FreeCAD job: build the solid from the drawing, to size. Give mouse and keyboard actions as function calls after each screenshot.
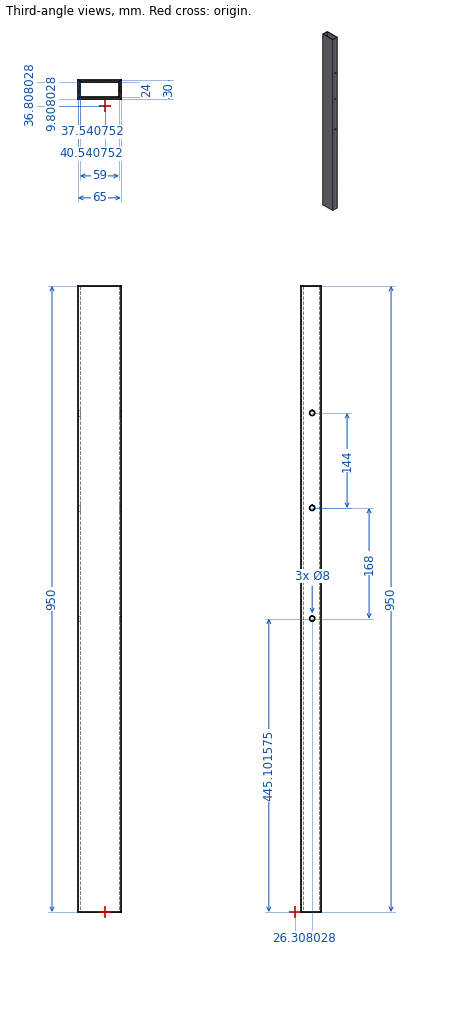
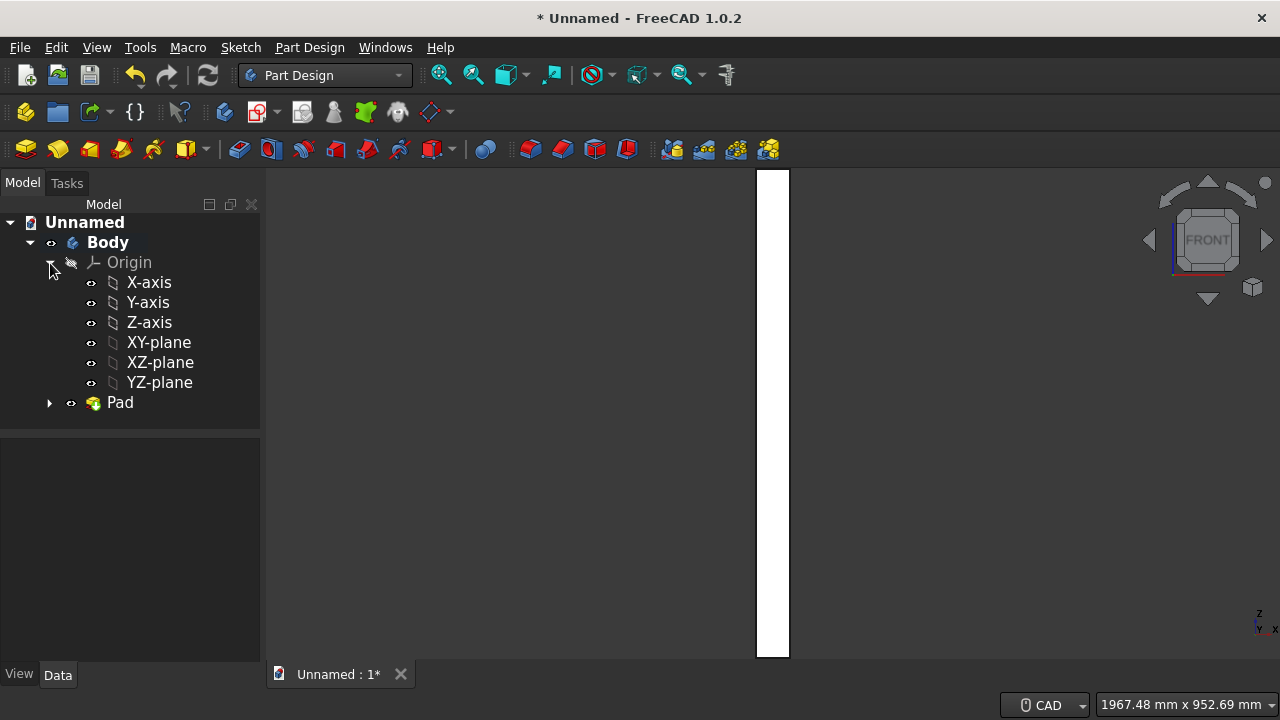
click(136, 343)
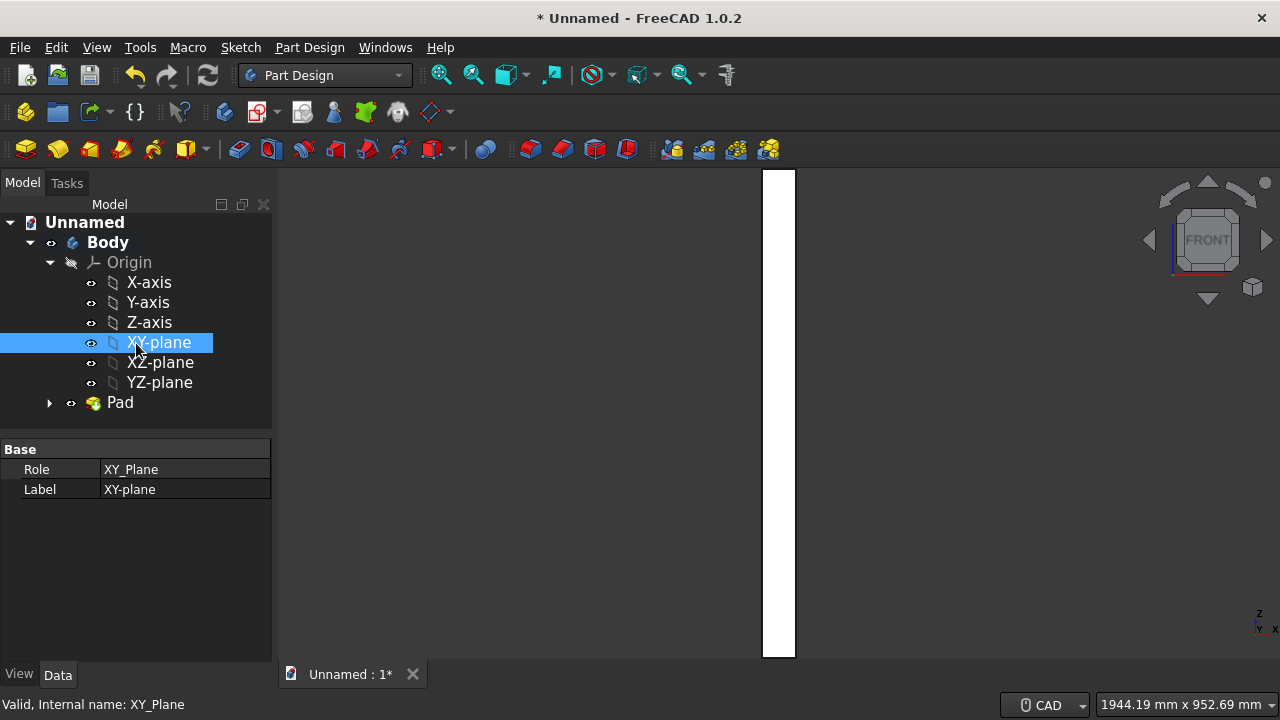
click(430, 112)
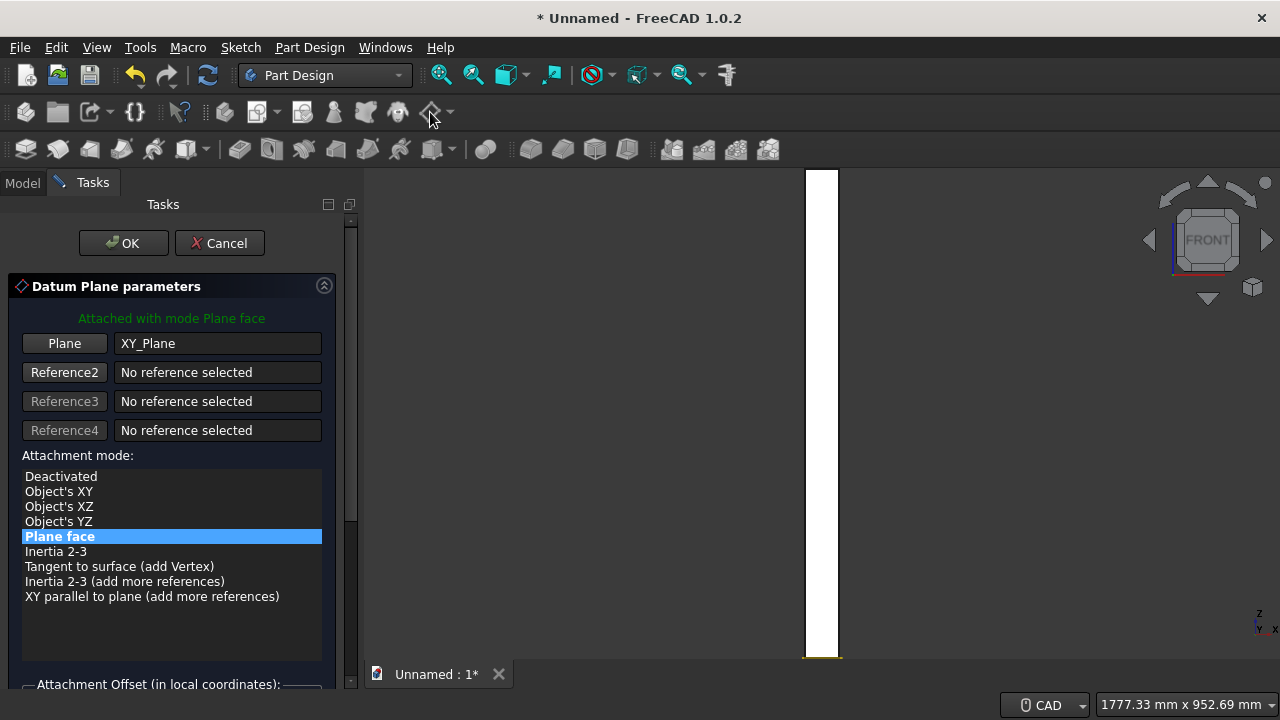
scroll(351, 451, down, 3)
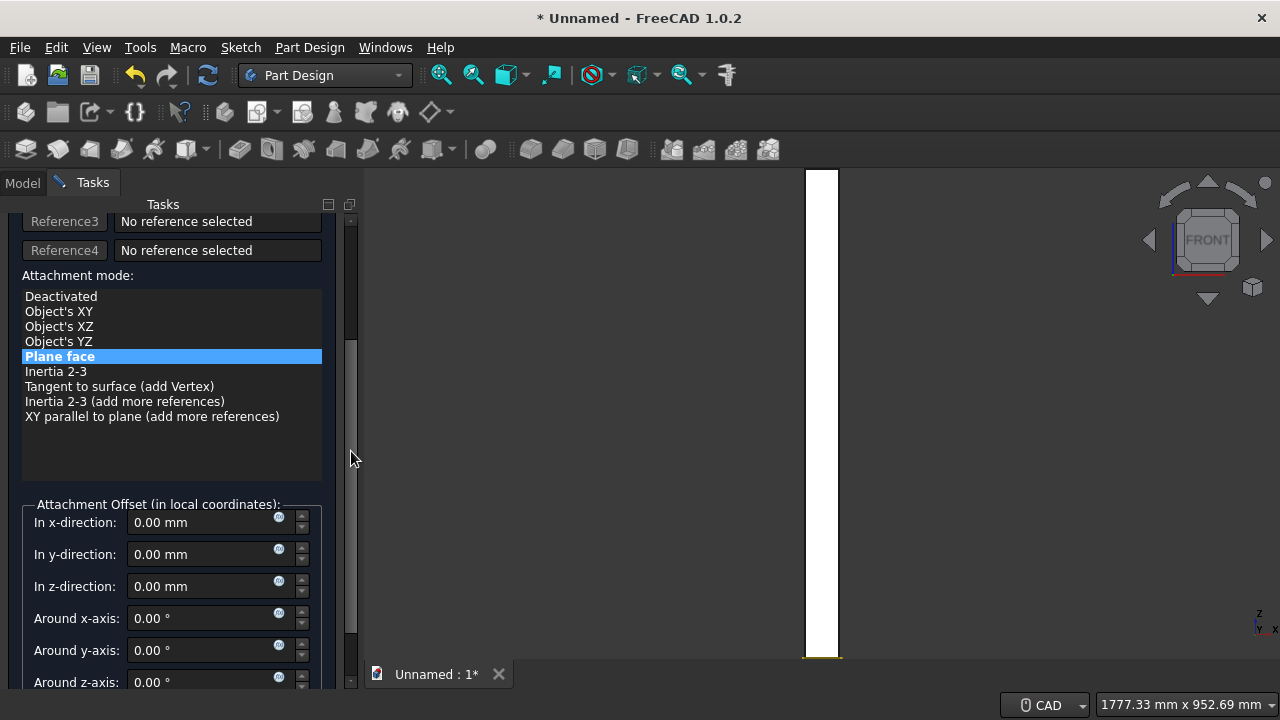
triple_click(210, 586)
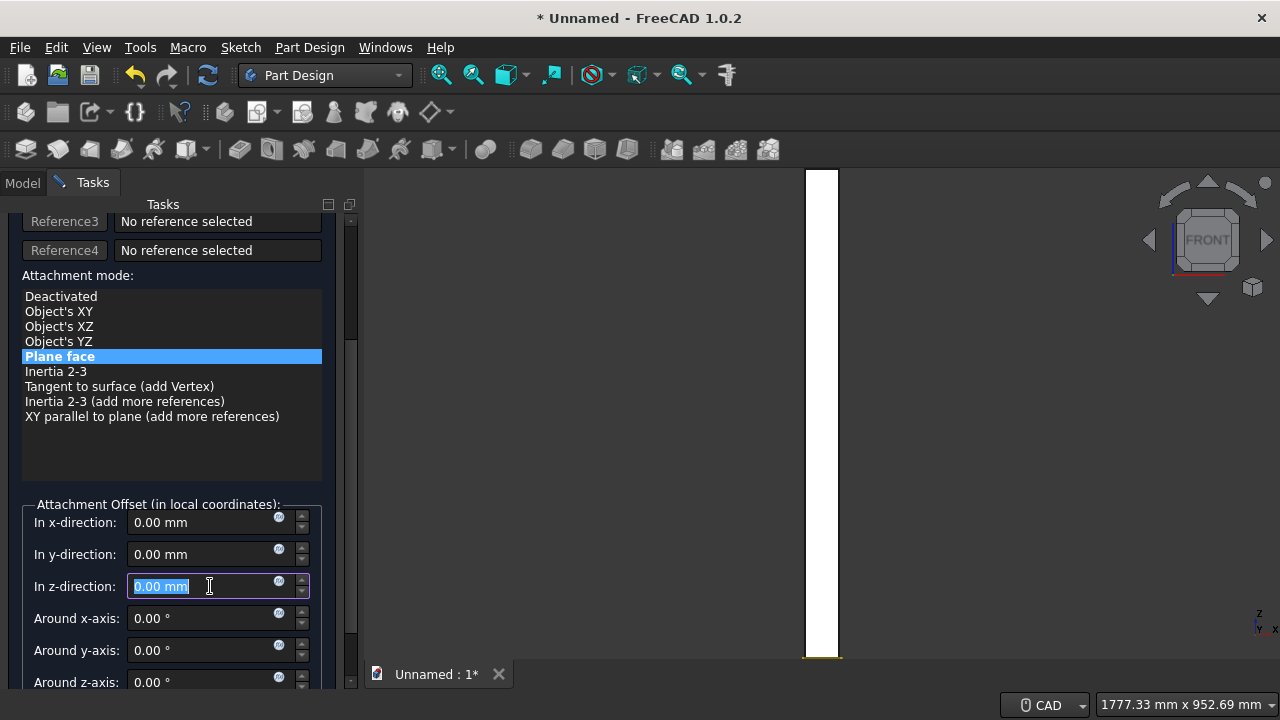
text(950)
key(Tab)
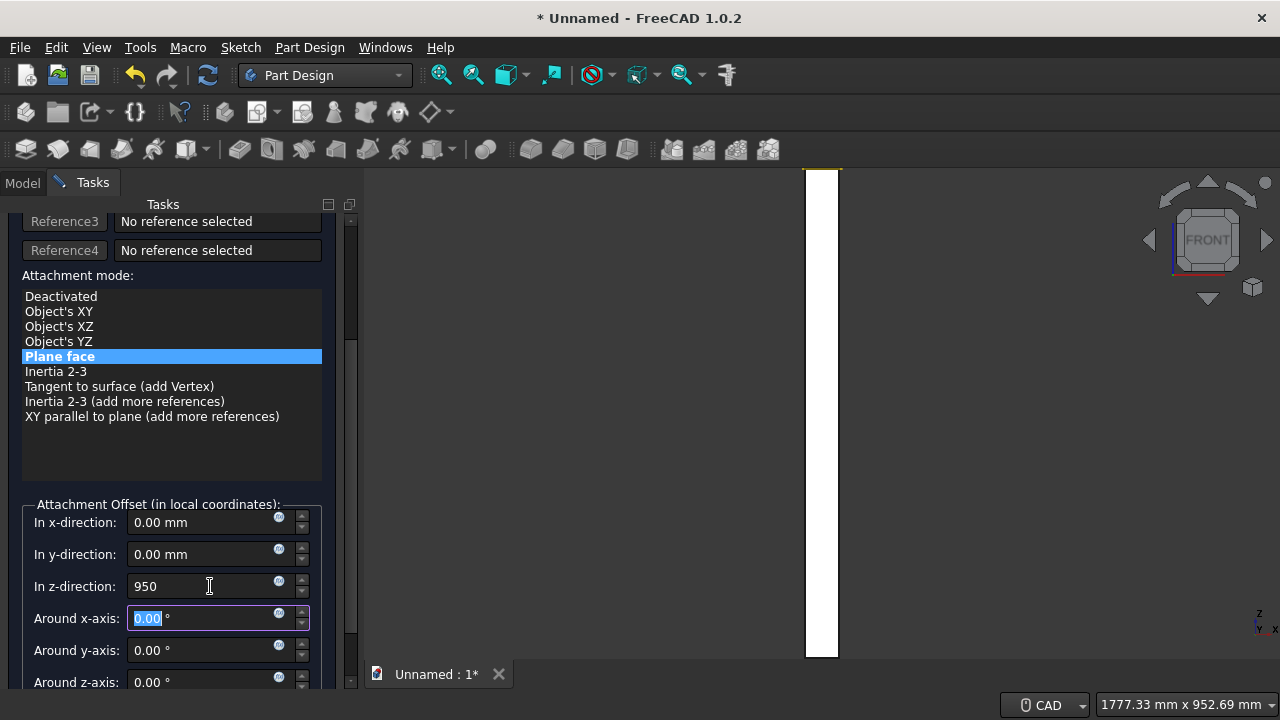
scroll(351, 451, up, 4)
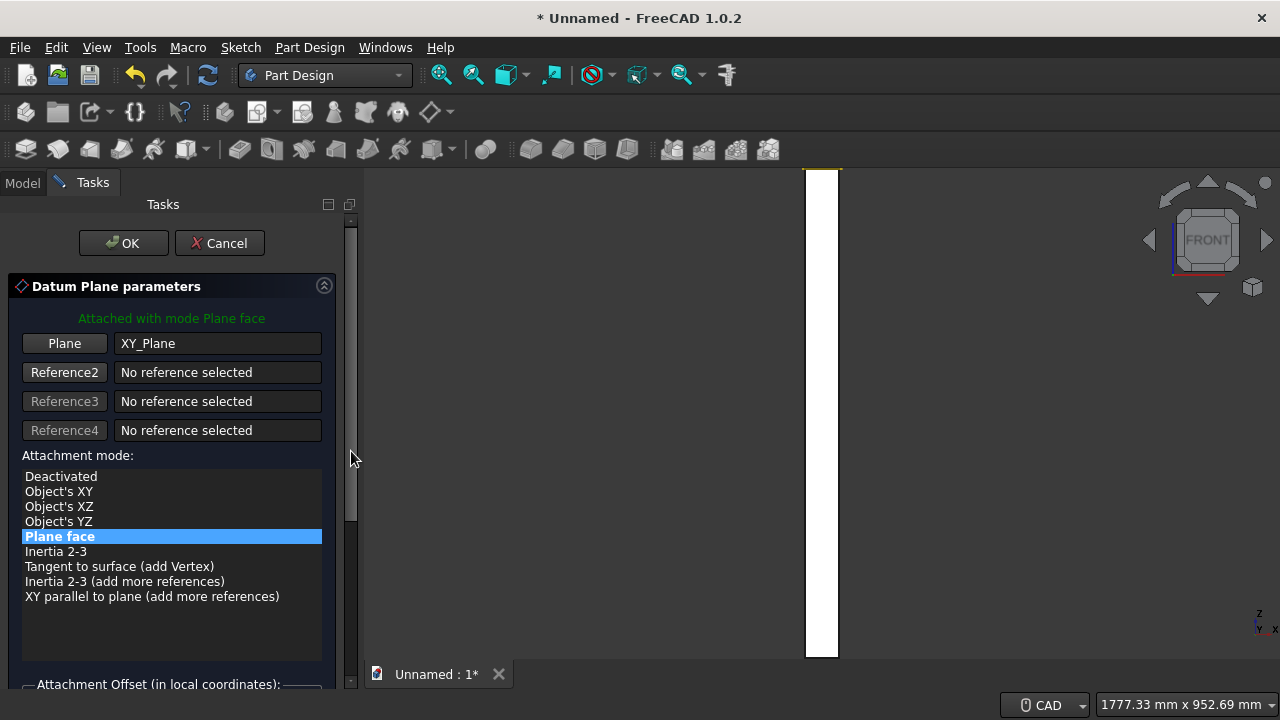
click(124, 243)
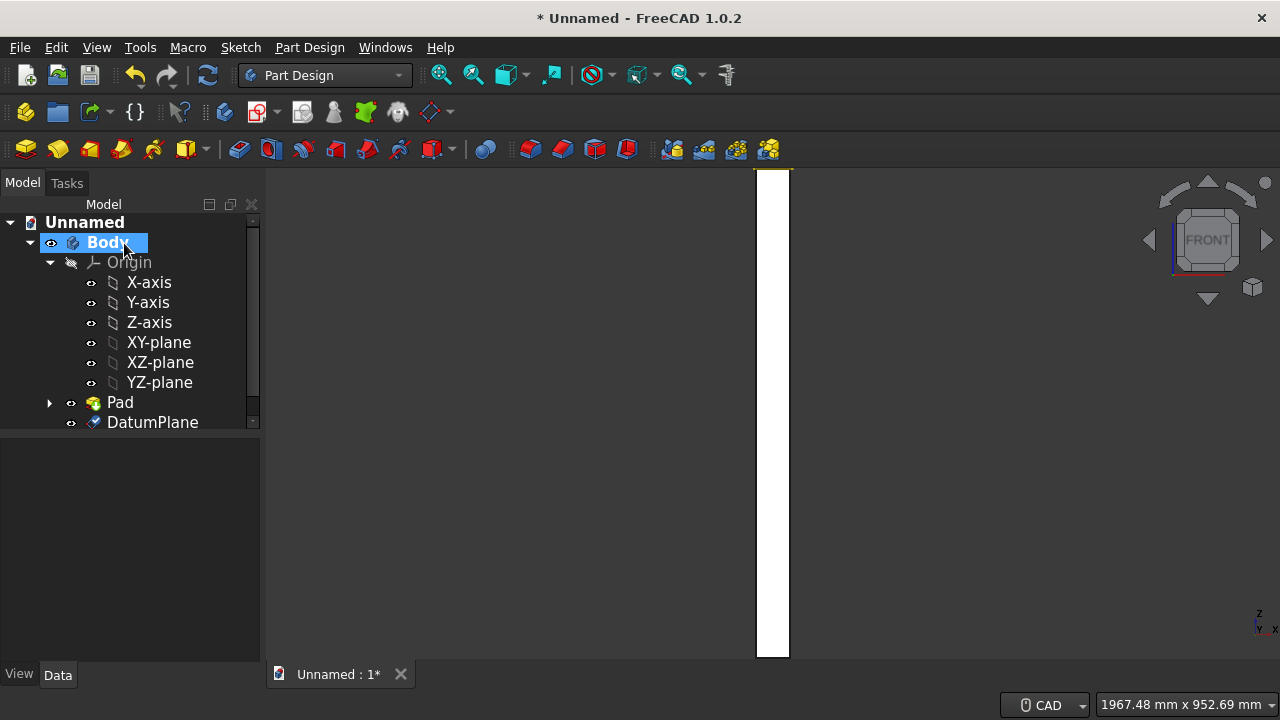
click(116, 423)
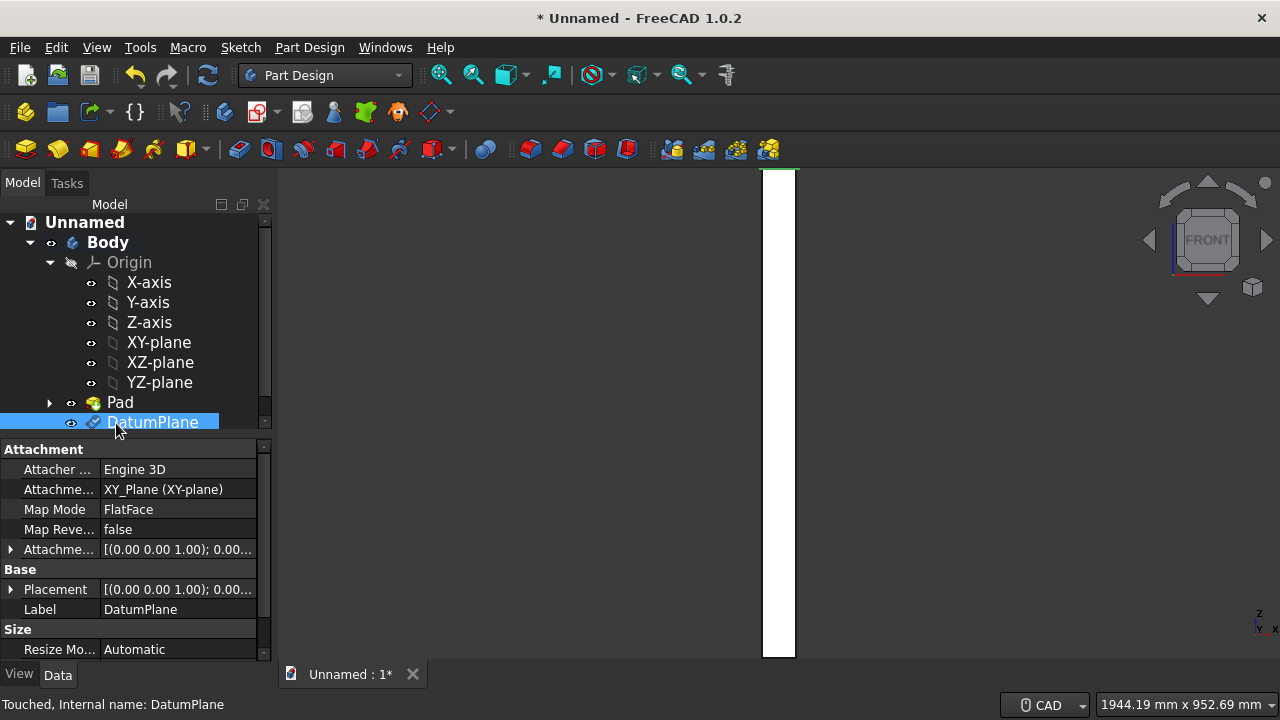
click(258, 112)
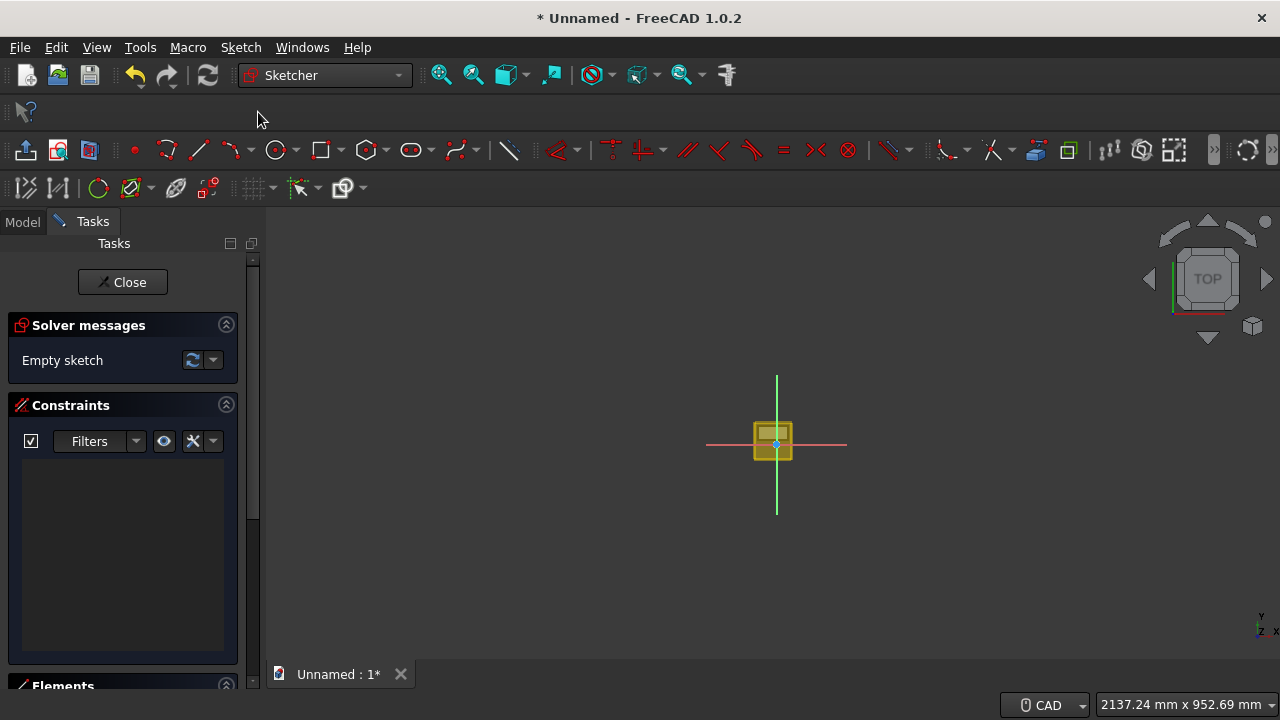
scroll(777, 436, up, 14)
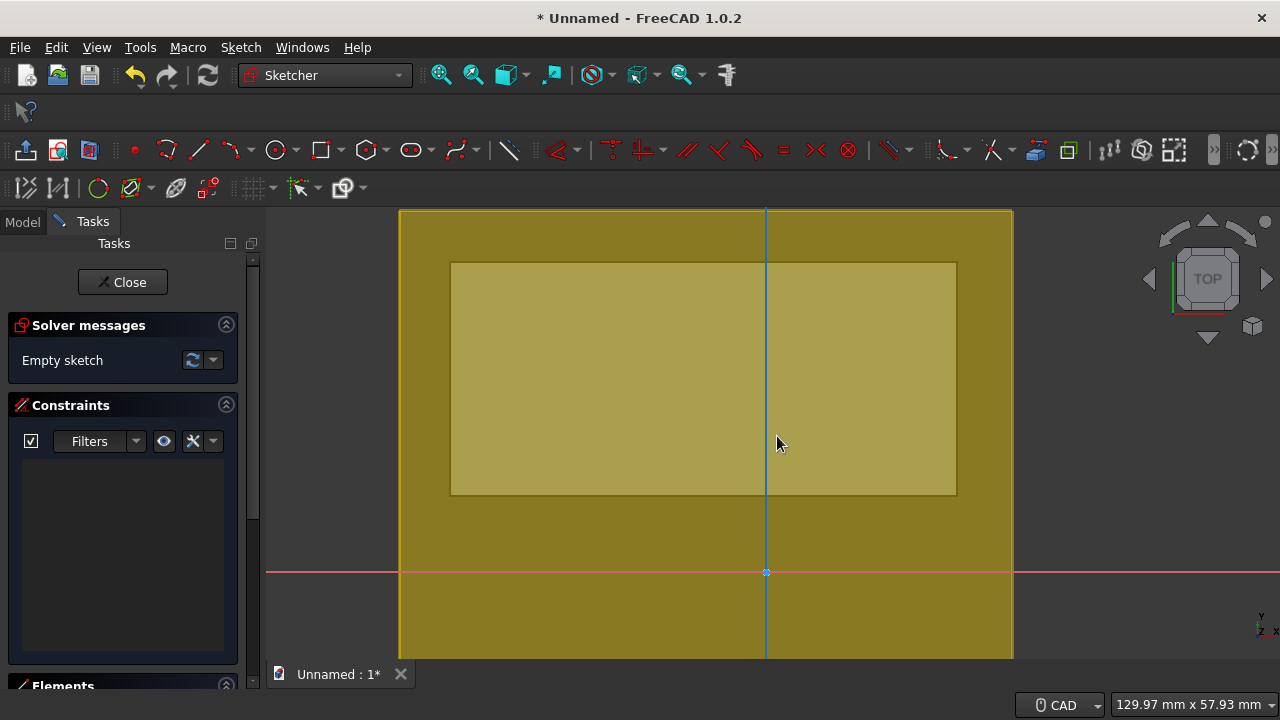
click(322, 150)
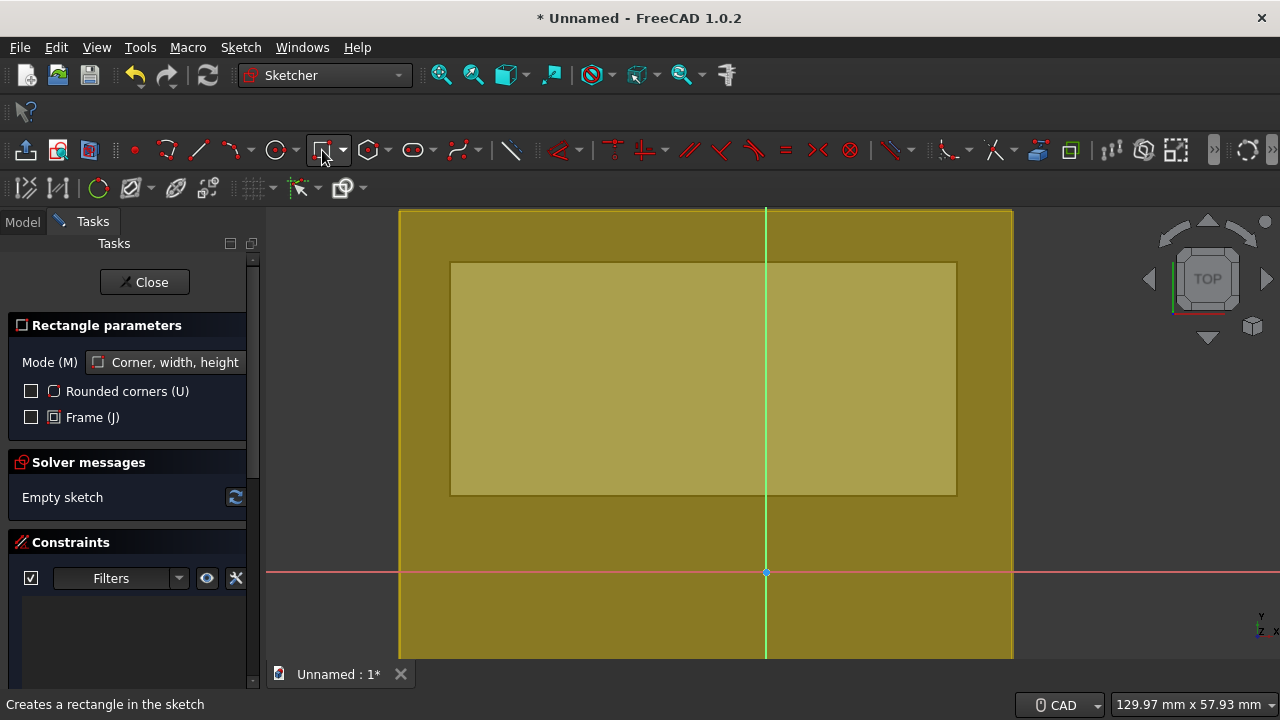
click(473, 285)
move(934, 472)